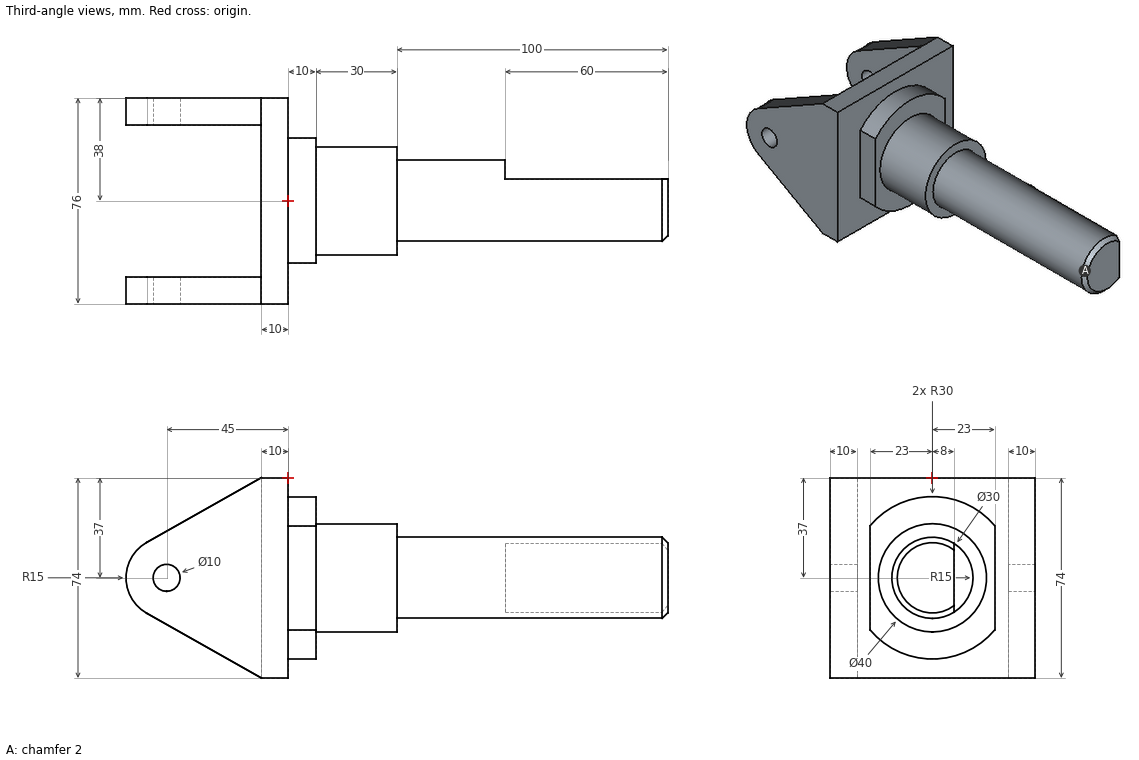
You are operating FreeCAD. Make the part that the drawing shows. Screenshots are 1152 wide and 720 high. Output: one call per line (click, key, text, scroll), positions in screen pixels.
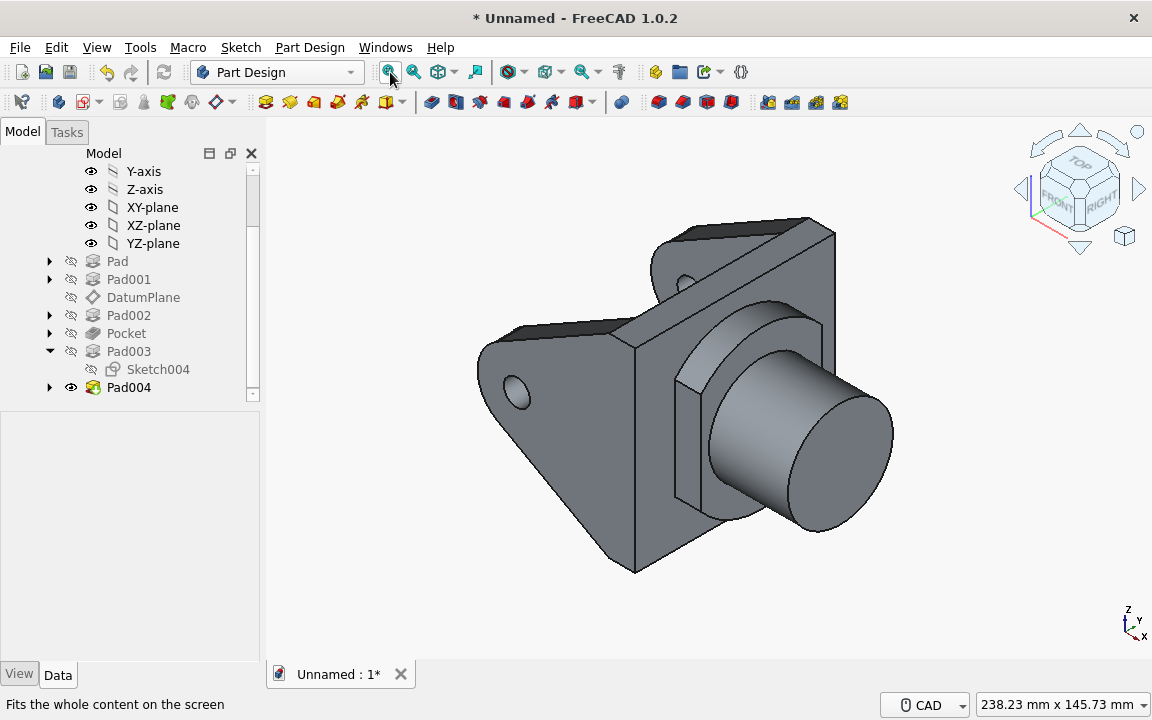
click(840, 463)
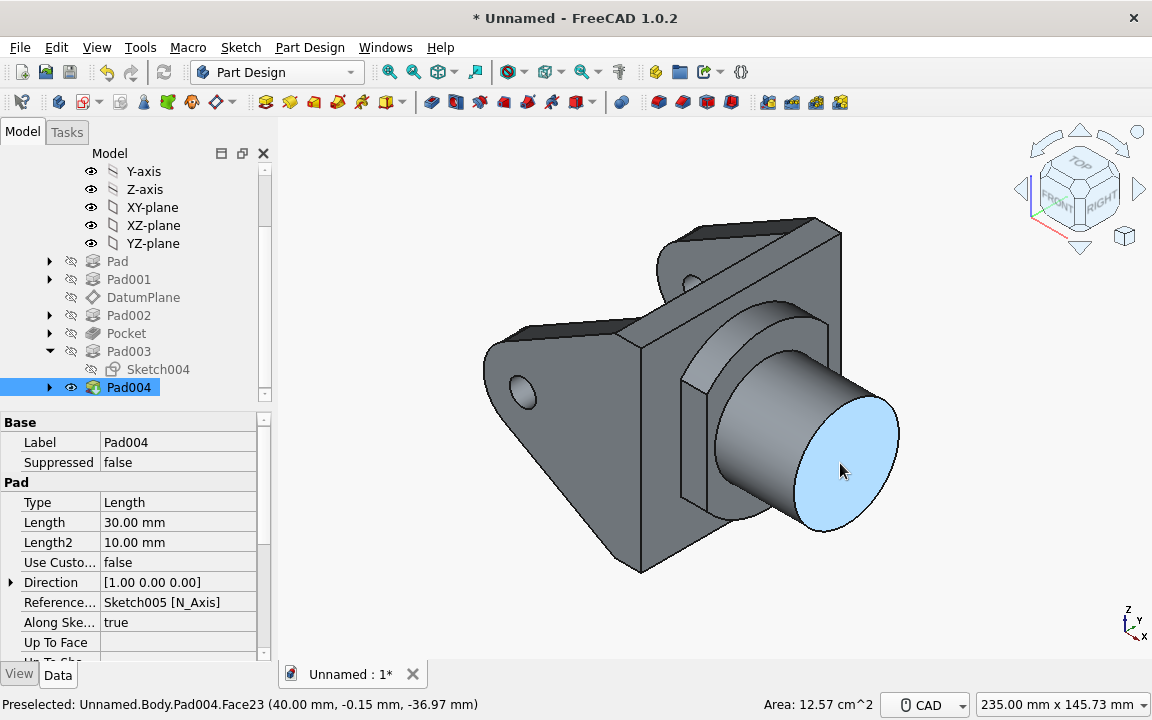
click(84, 102)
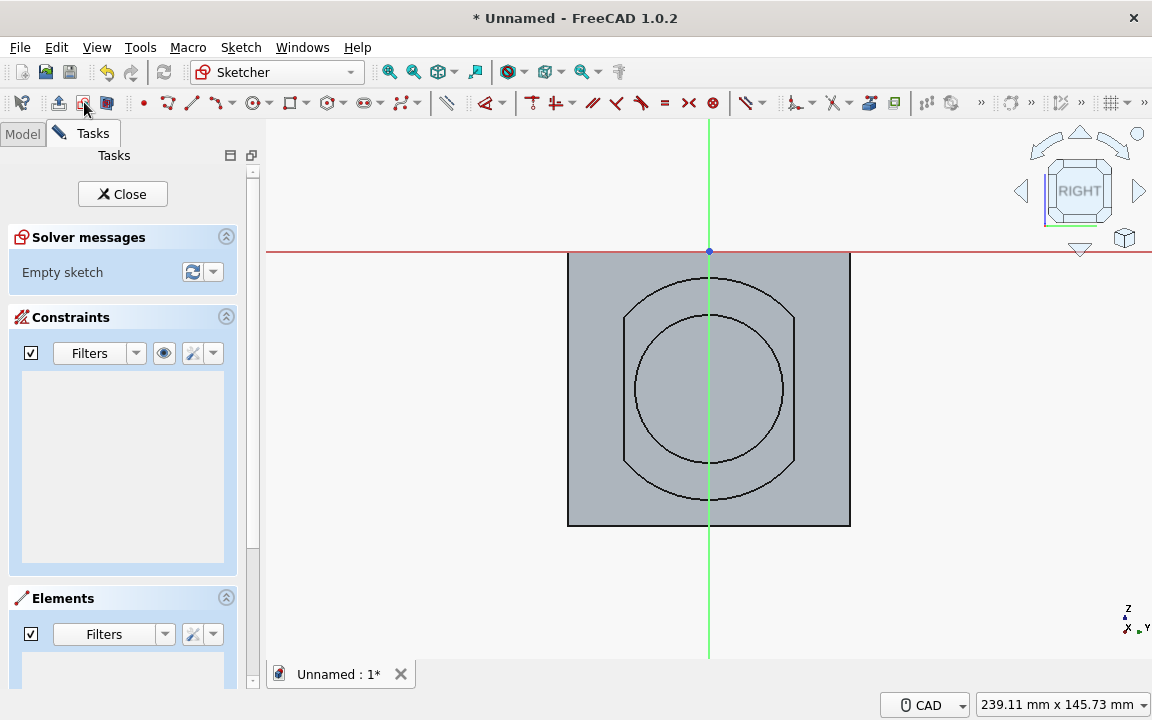
scroll(792, 299, up, 3)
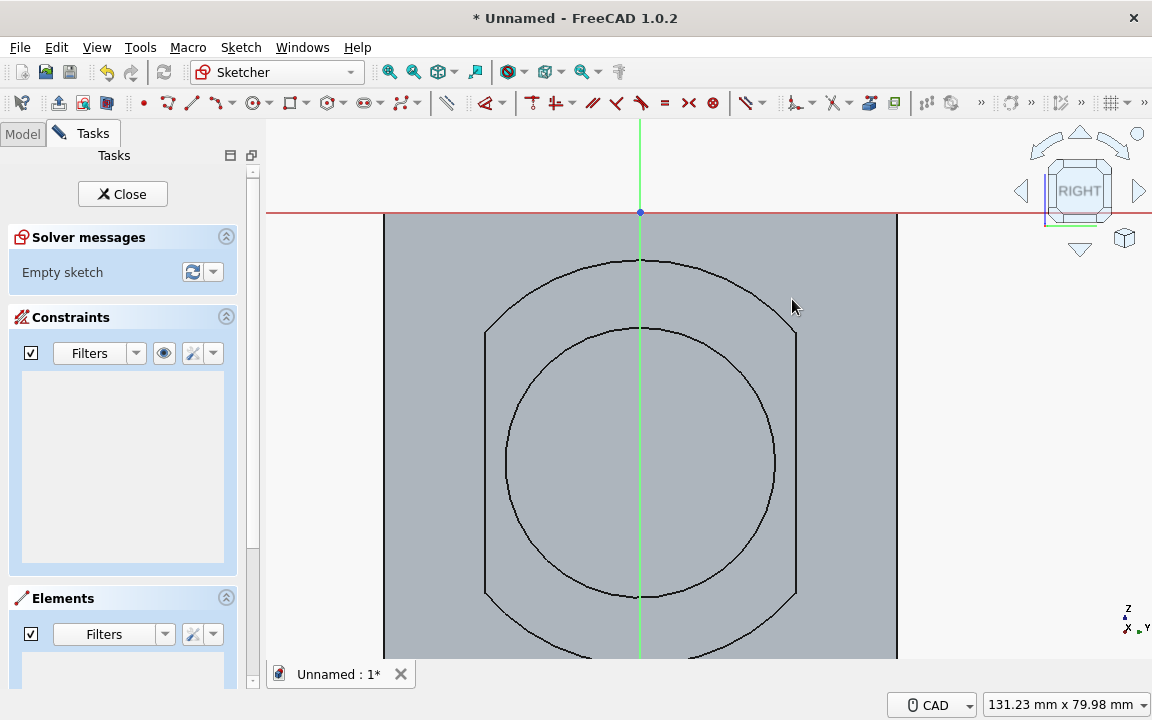
click(254, 104)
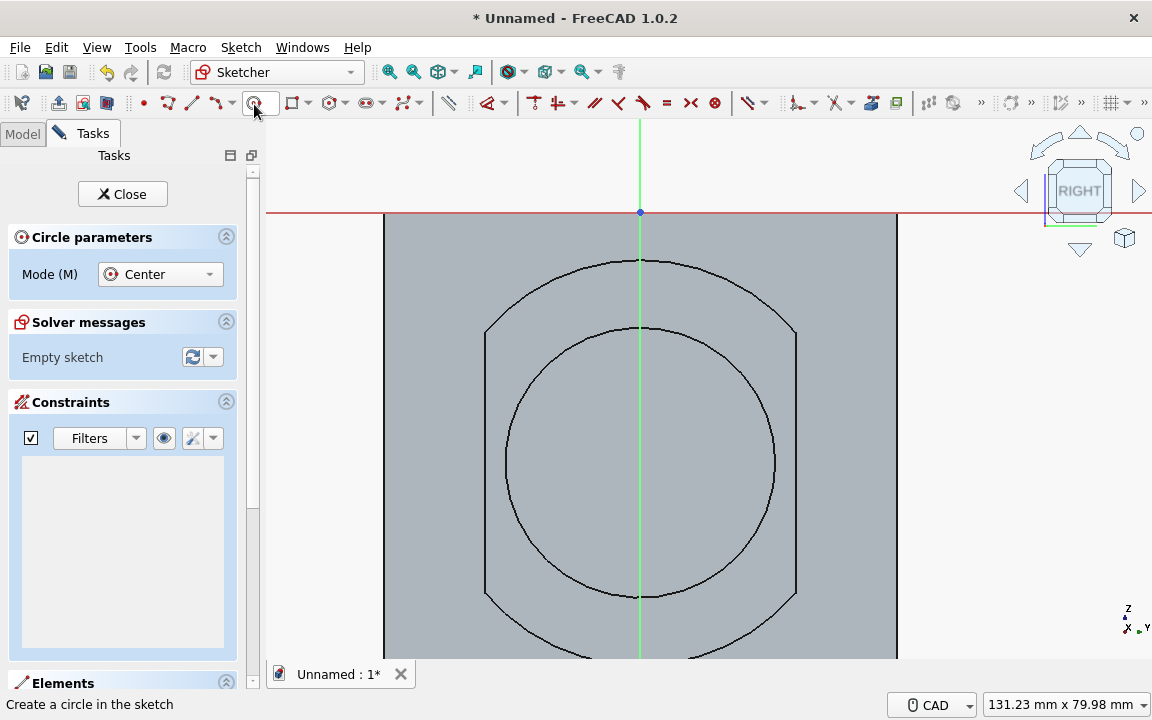
click(640, 463)
click(712, 391)
key(Escape)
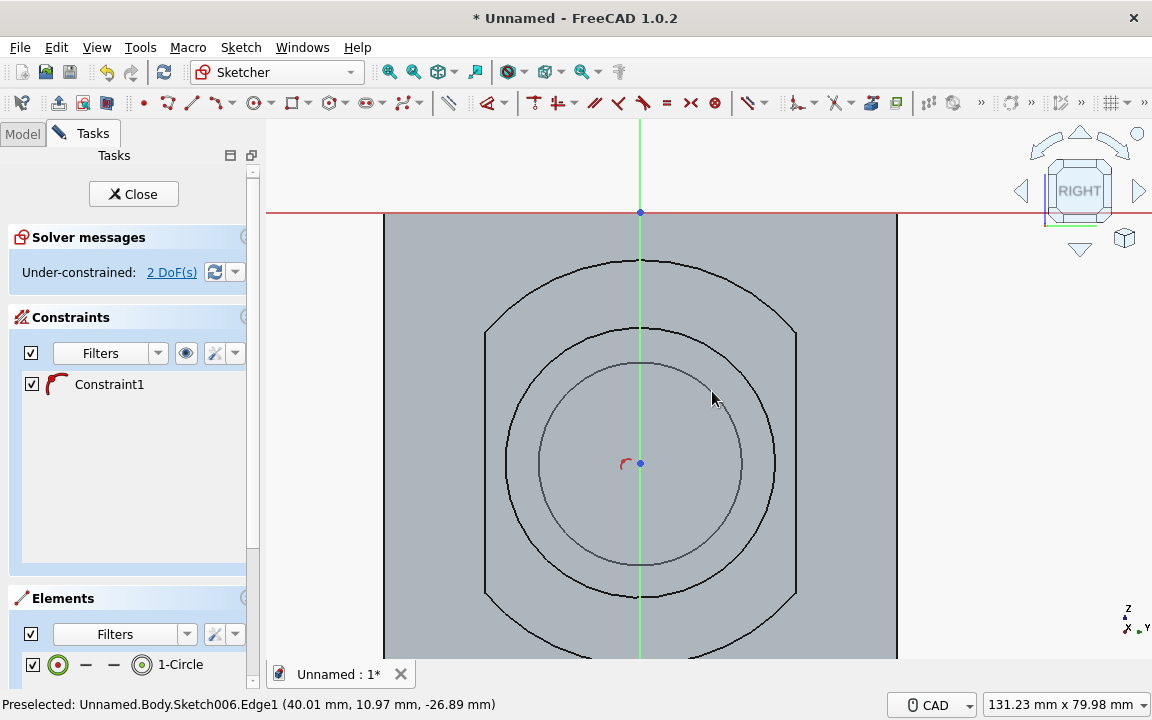
click(488, 104)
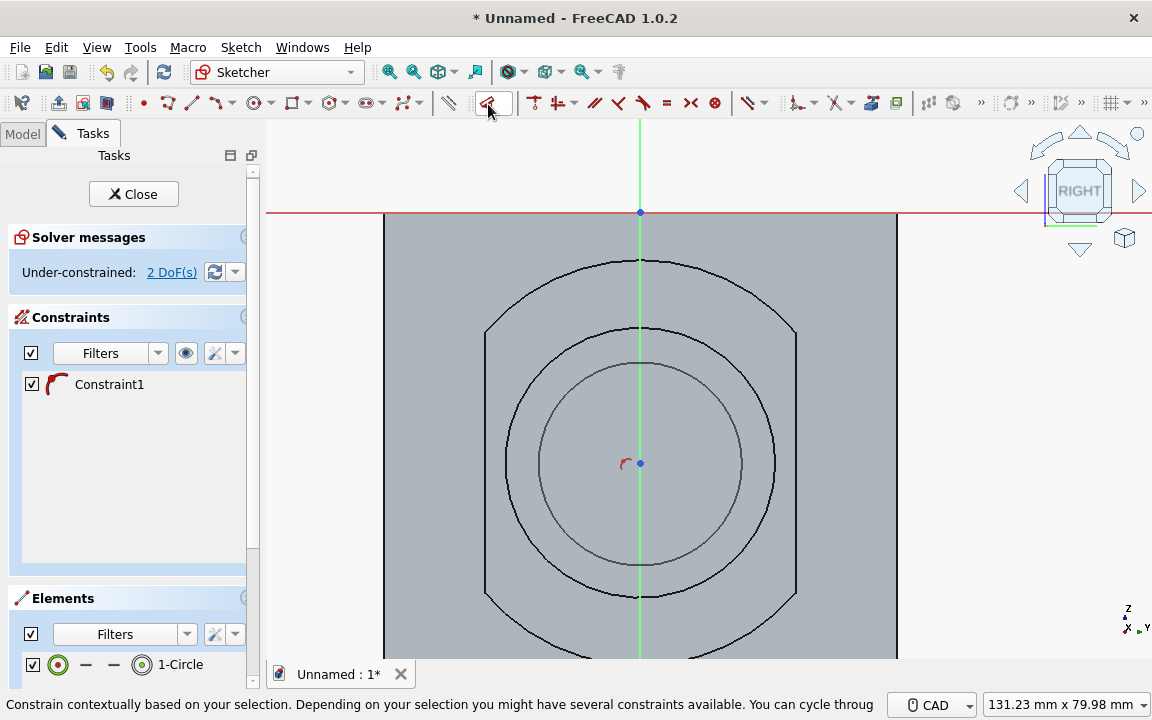
click(712, 392)
click(735, 369)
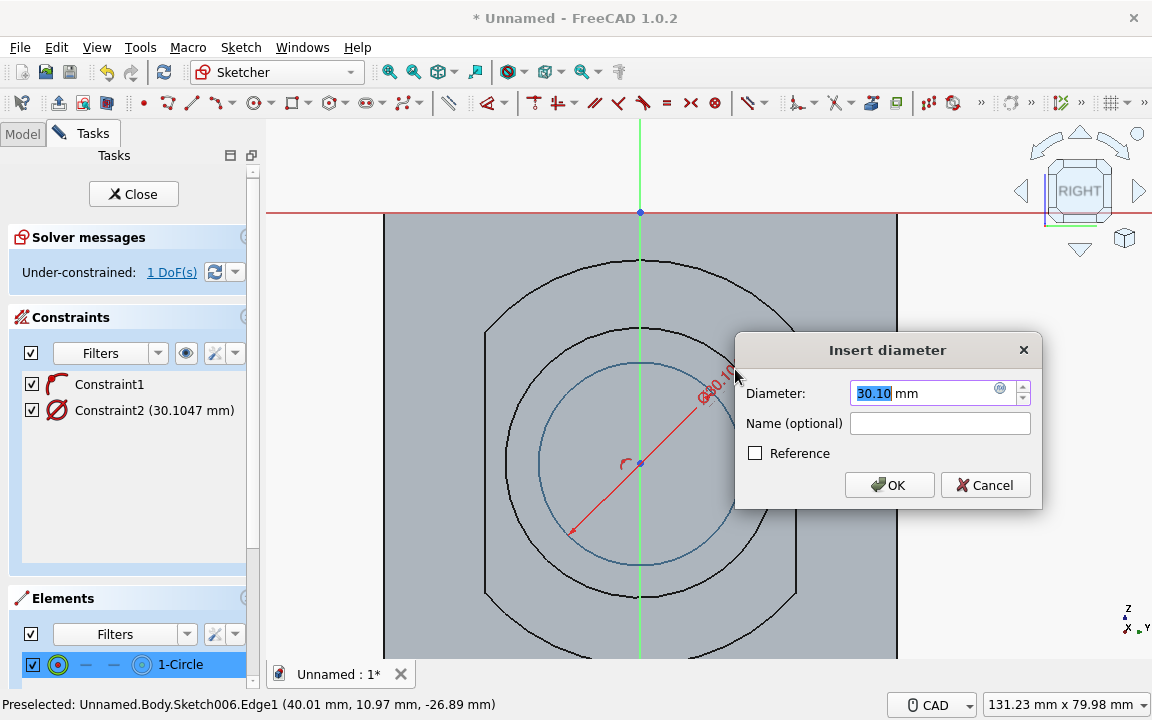
text(30)
key(Return)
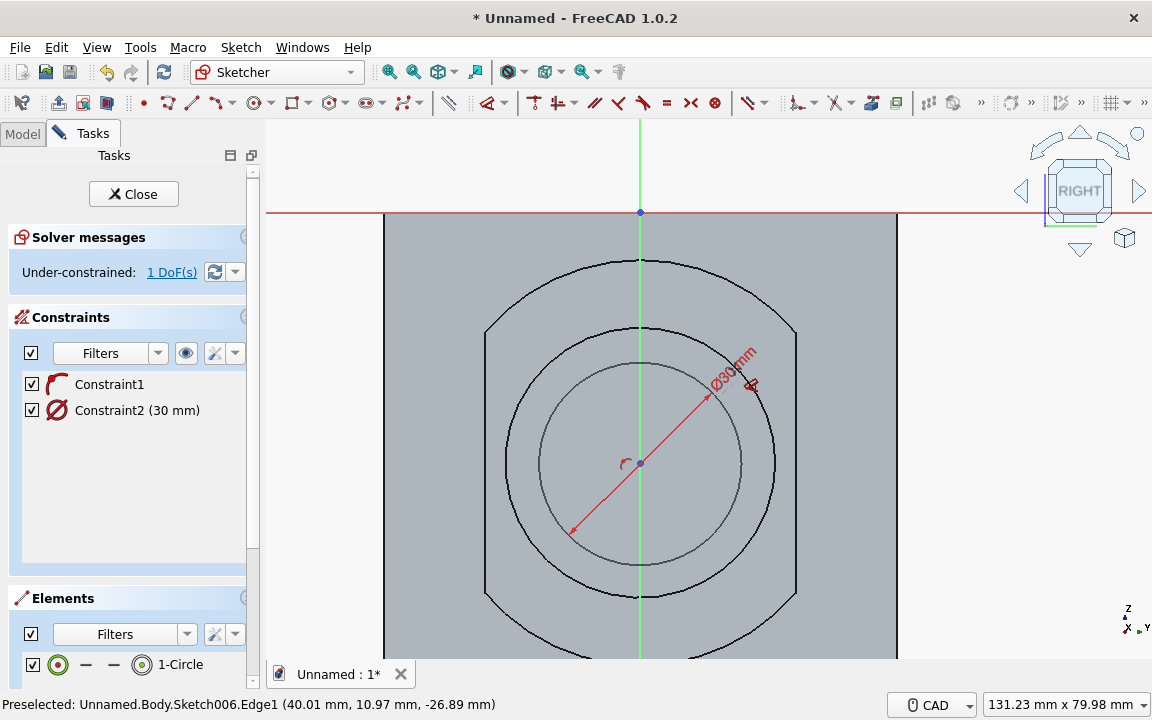
click(640, 464)
click(674, 338)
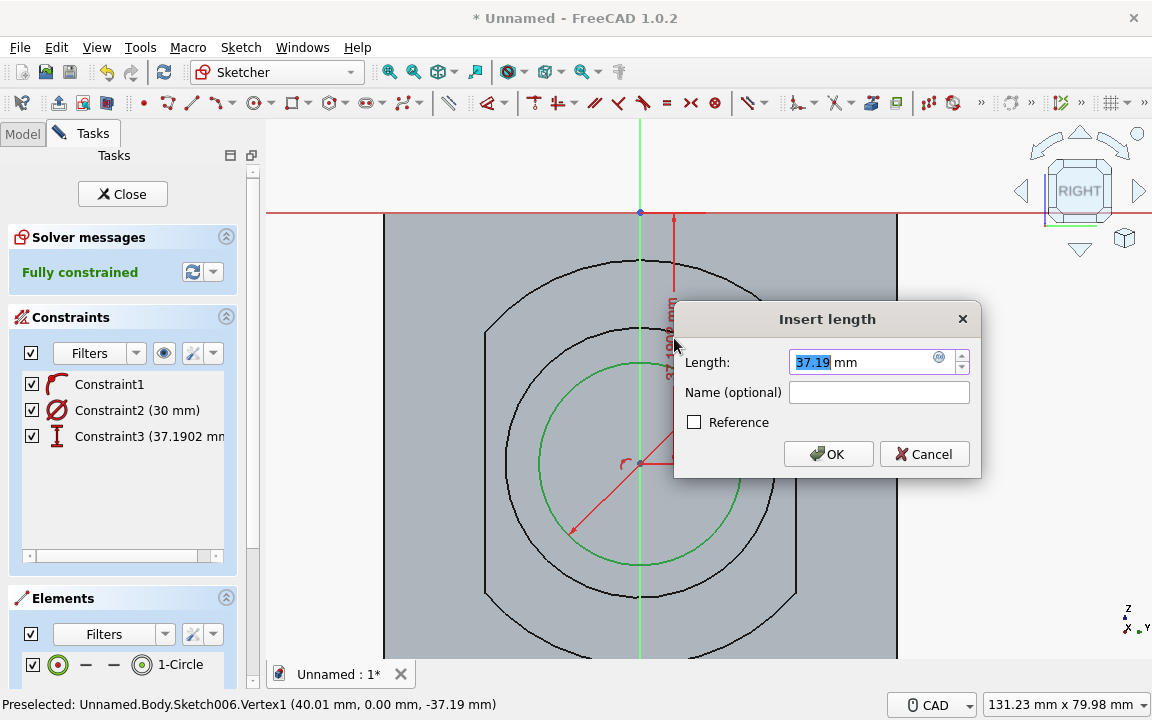
text(37)
key(Return)
key(Escape)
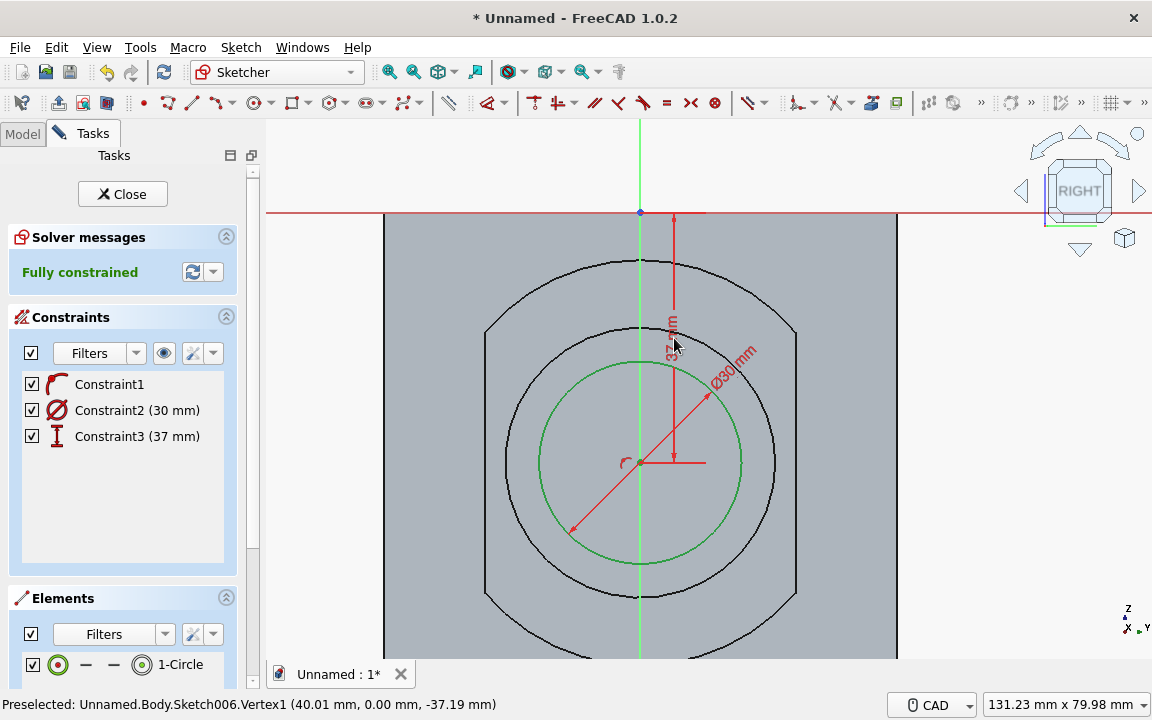
click(123, 194)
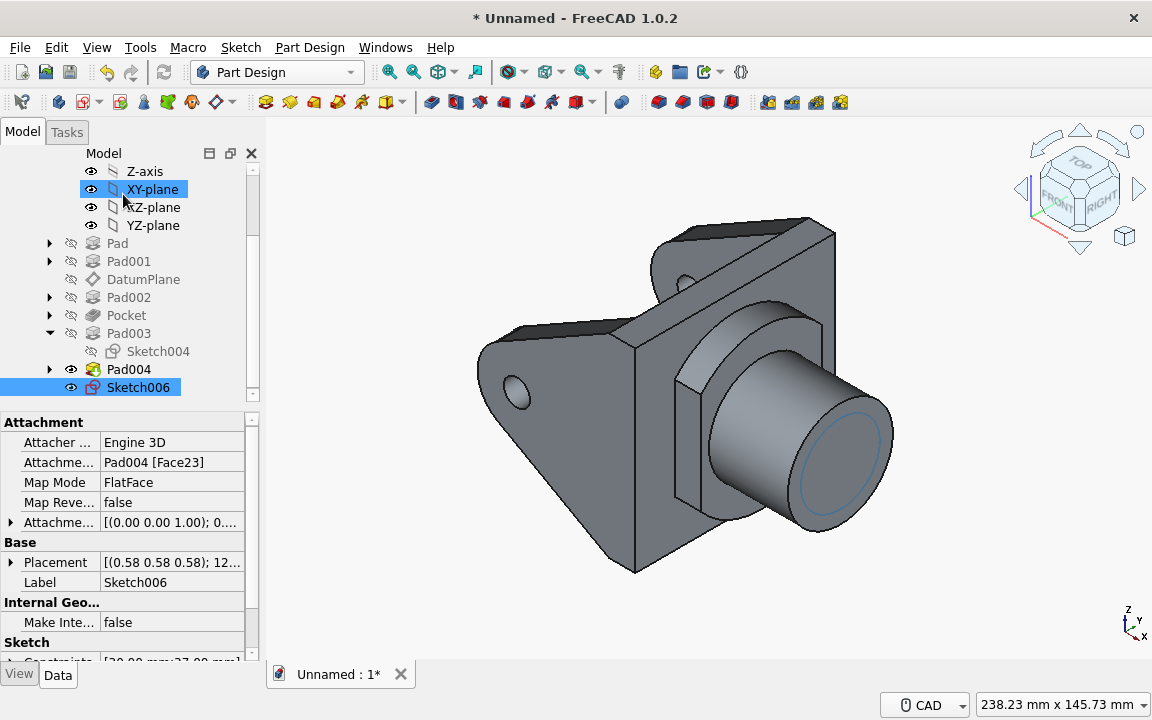
click(266, 102)